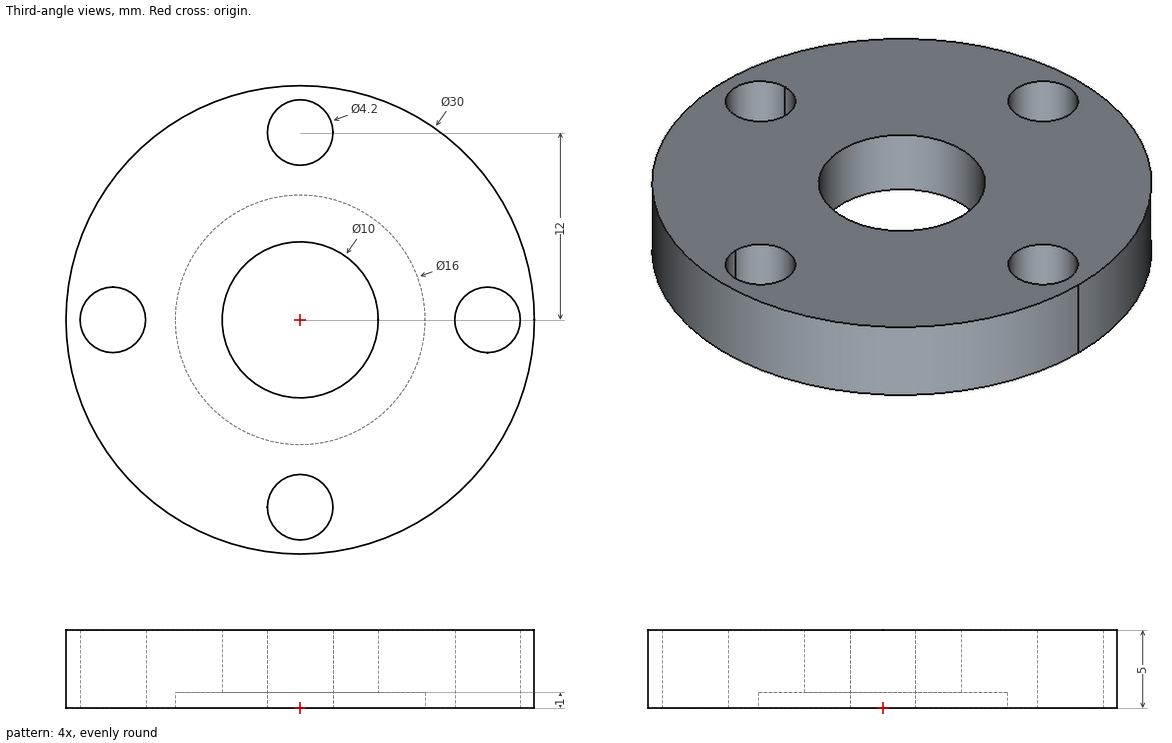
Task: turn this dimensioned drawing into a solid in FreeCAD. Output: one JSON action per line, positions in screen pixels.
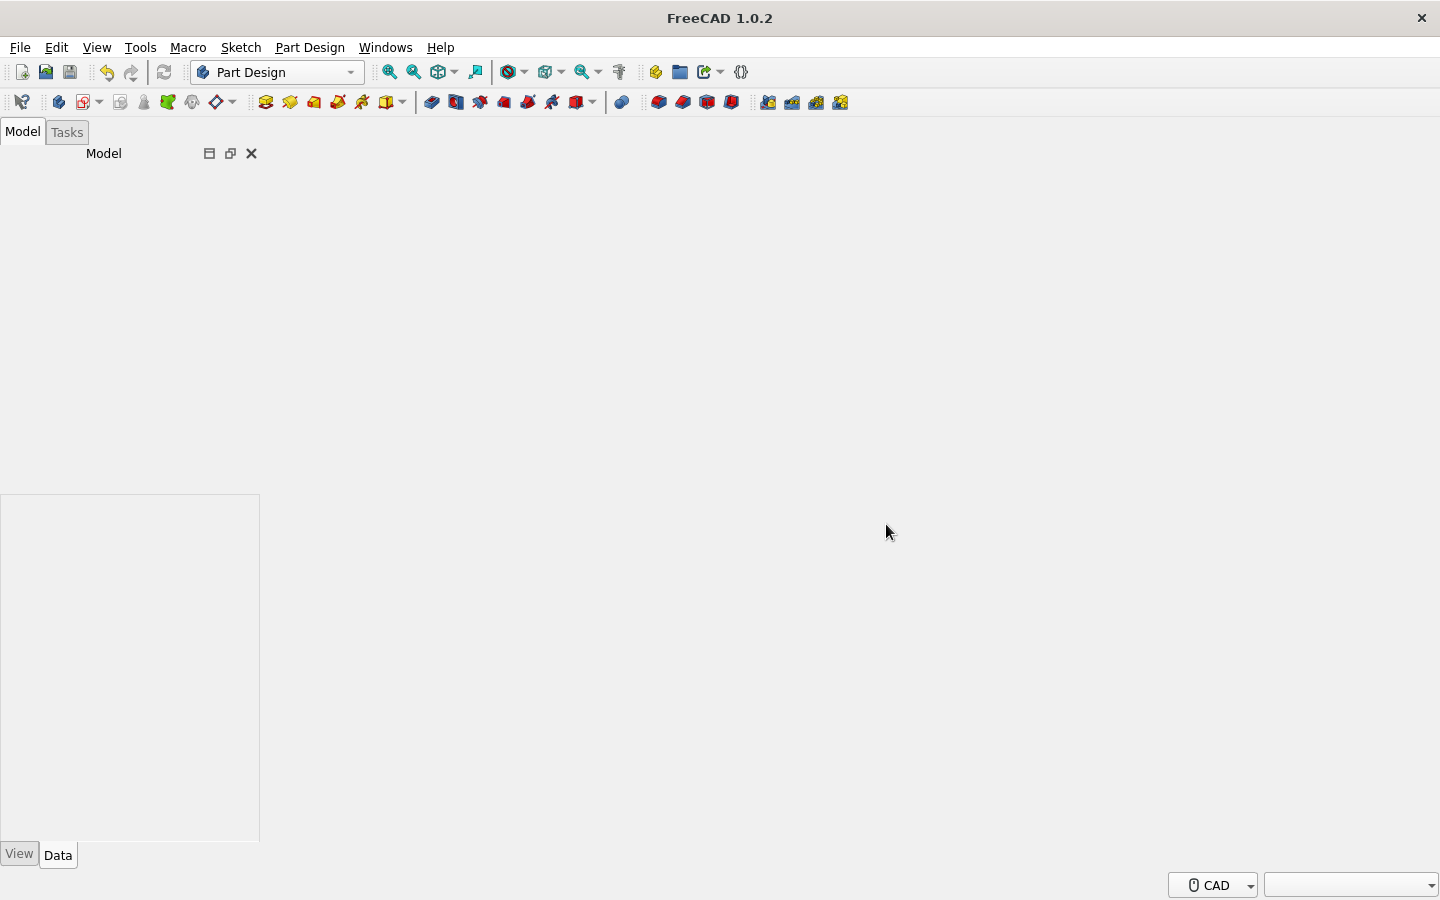
{"action": "left_click", "coordinate": [22, 72]}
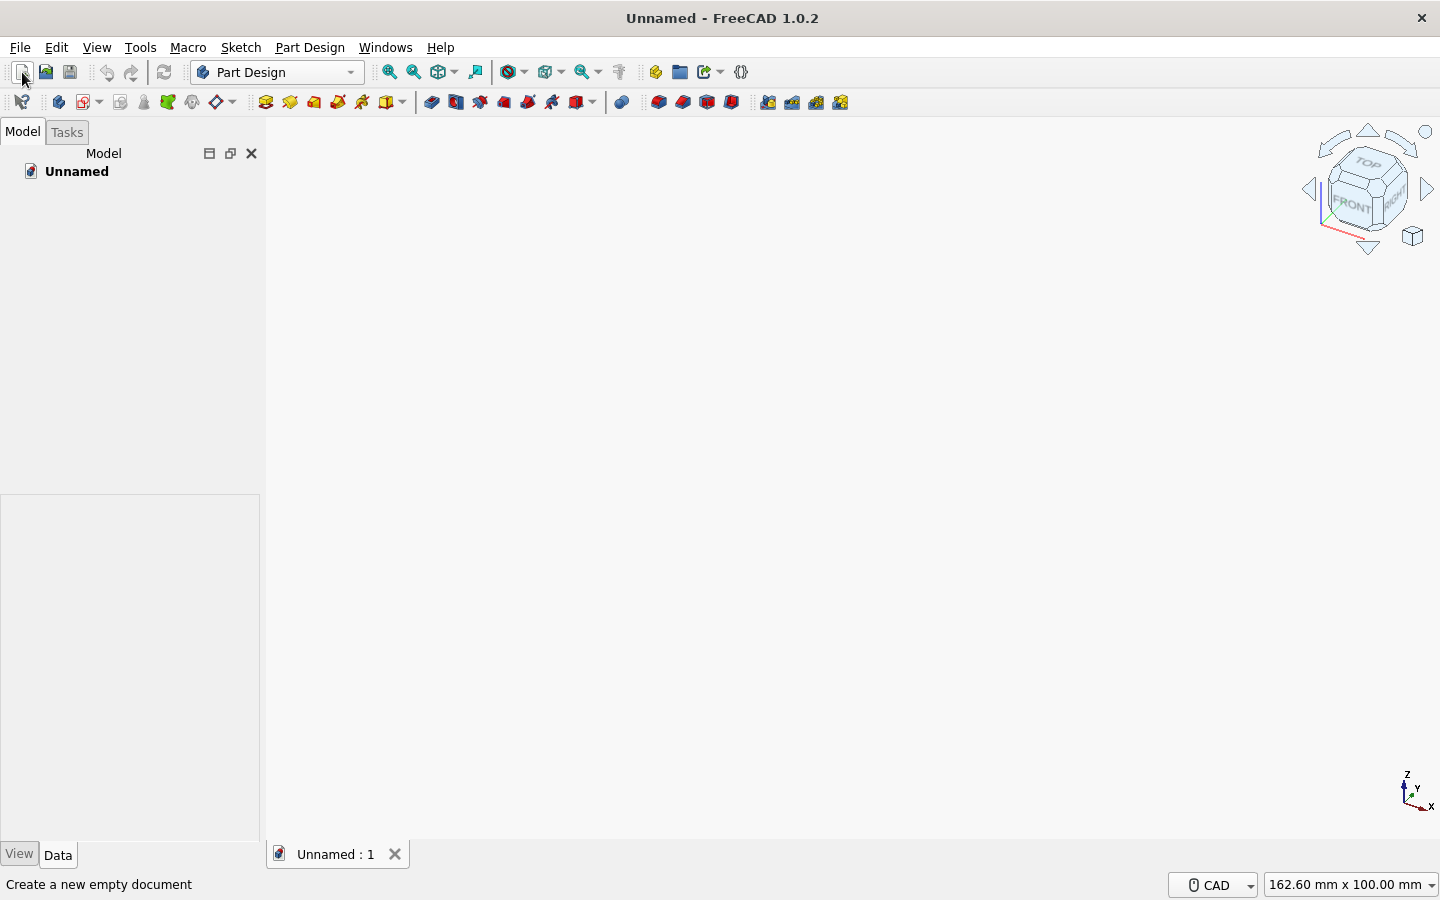
{"action": "left_click", "coordinate": [84, 102]}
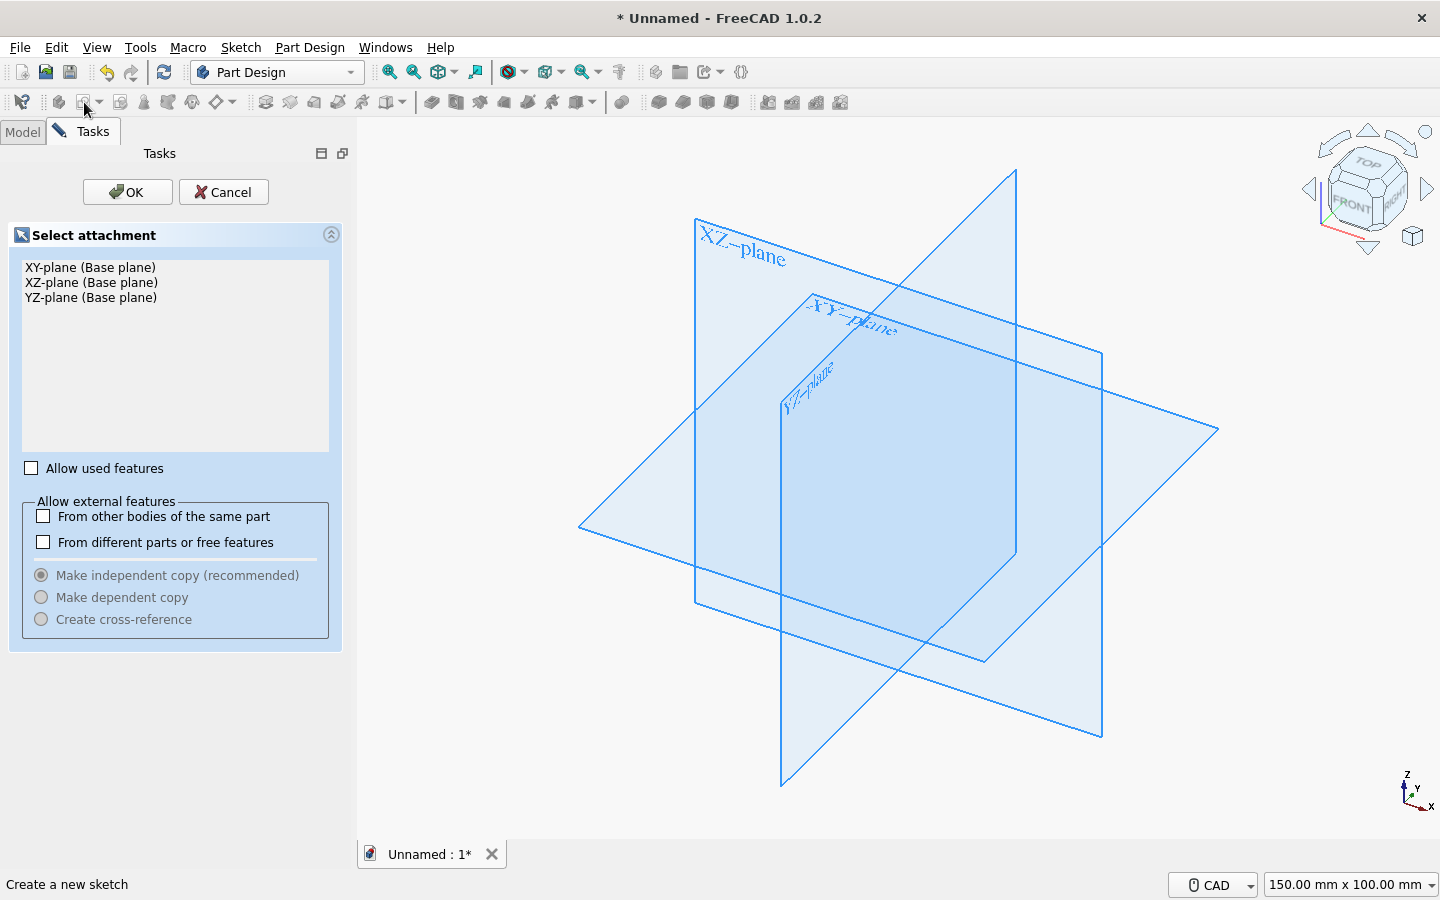
{"action": "left_click", "coordinate": [82, 268]}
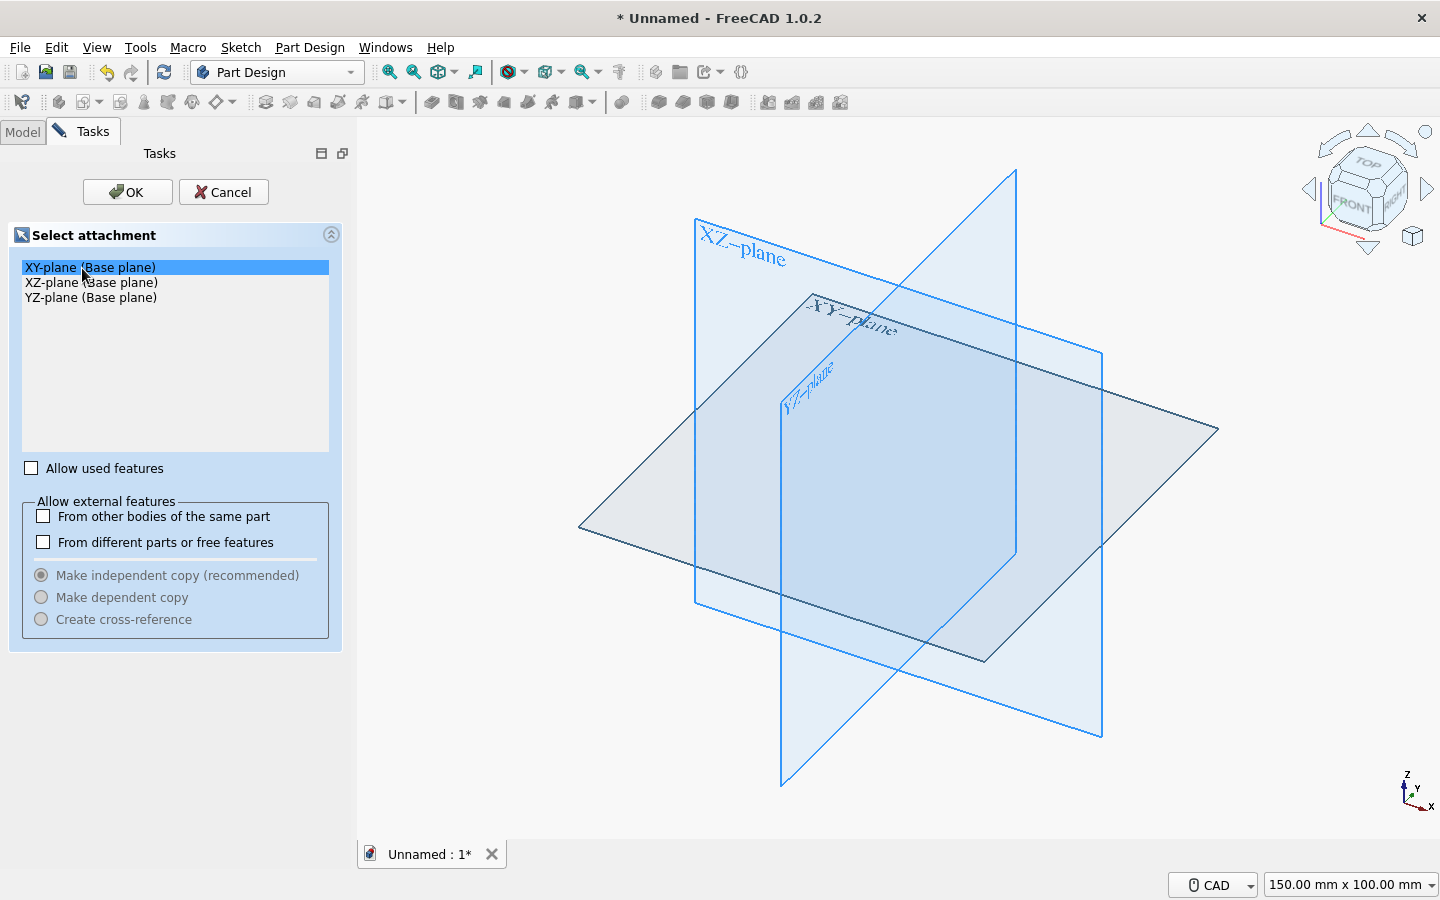
{"action": "left_click", "coordinate": [128, 192]}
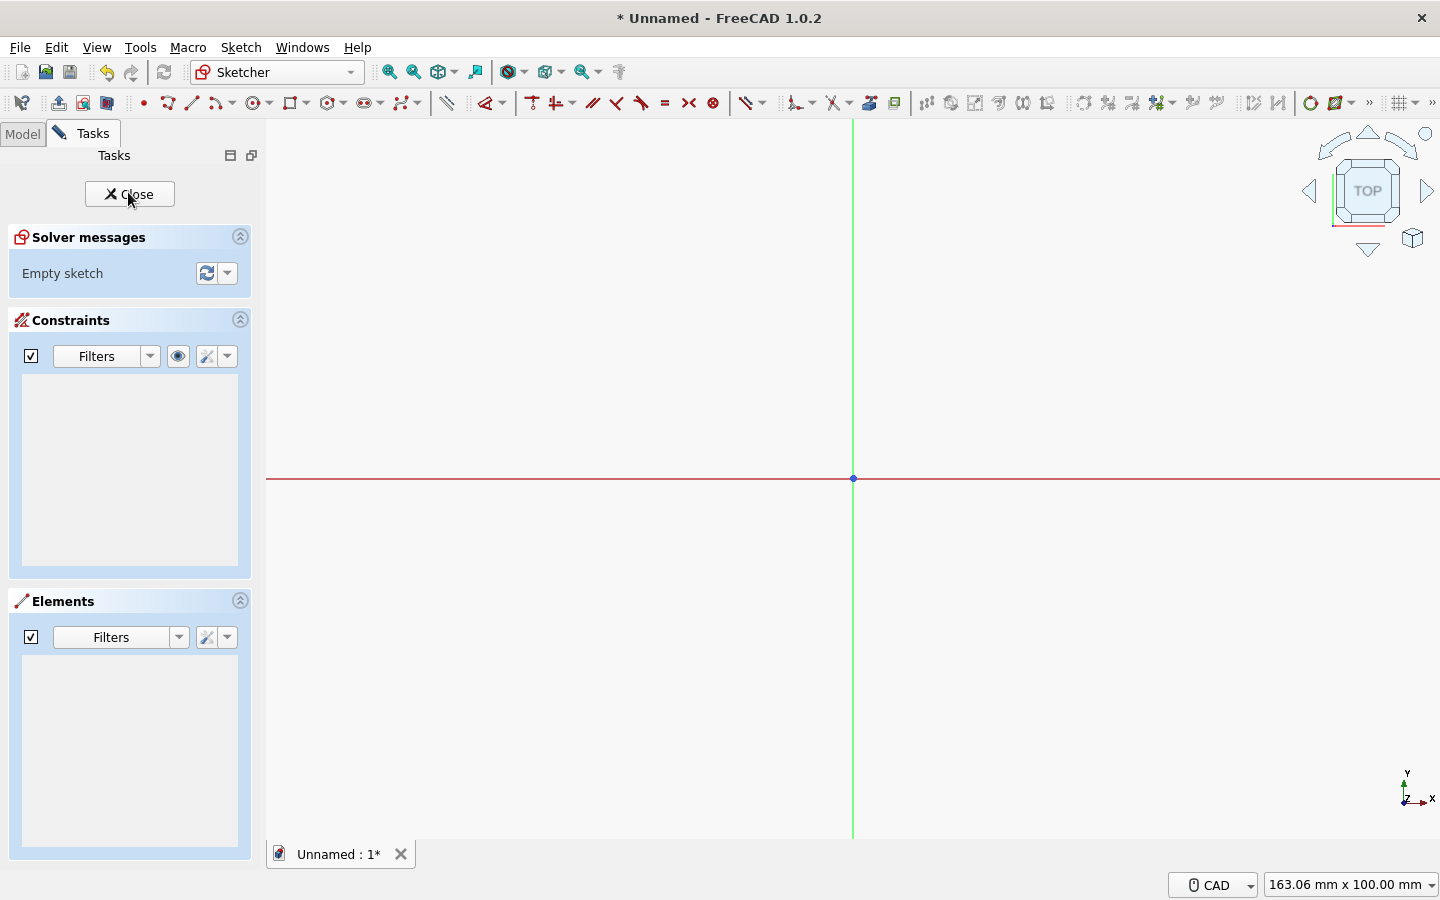
{"action": "scroll", "coordinate": [909, 479], "scroll_direction": "up", "scroll_amount": 4}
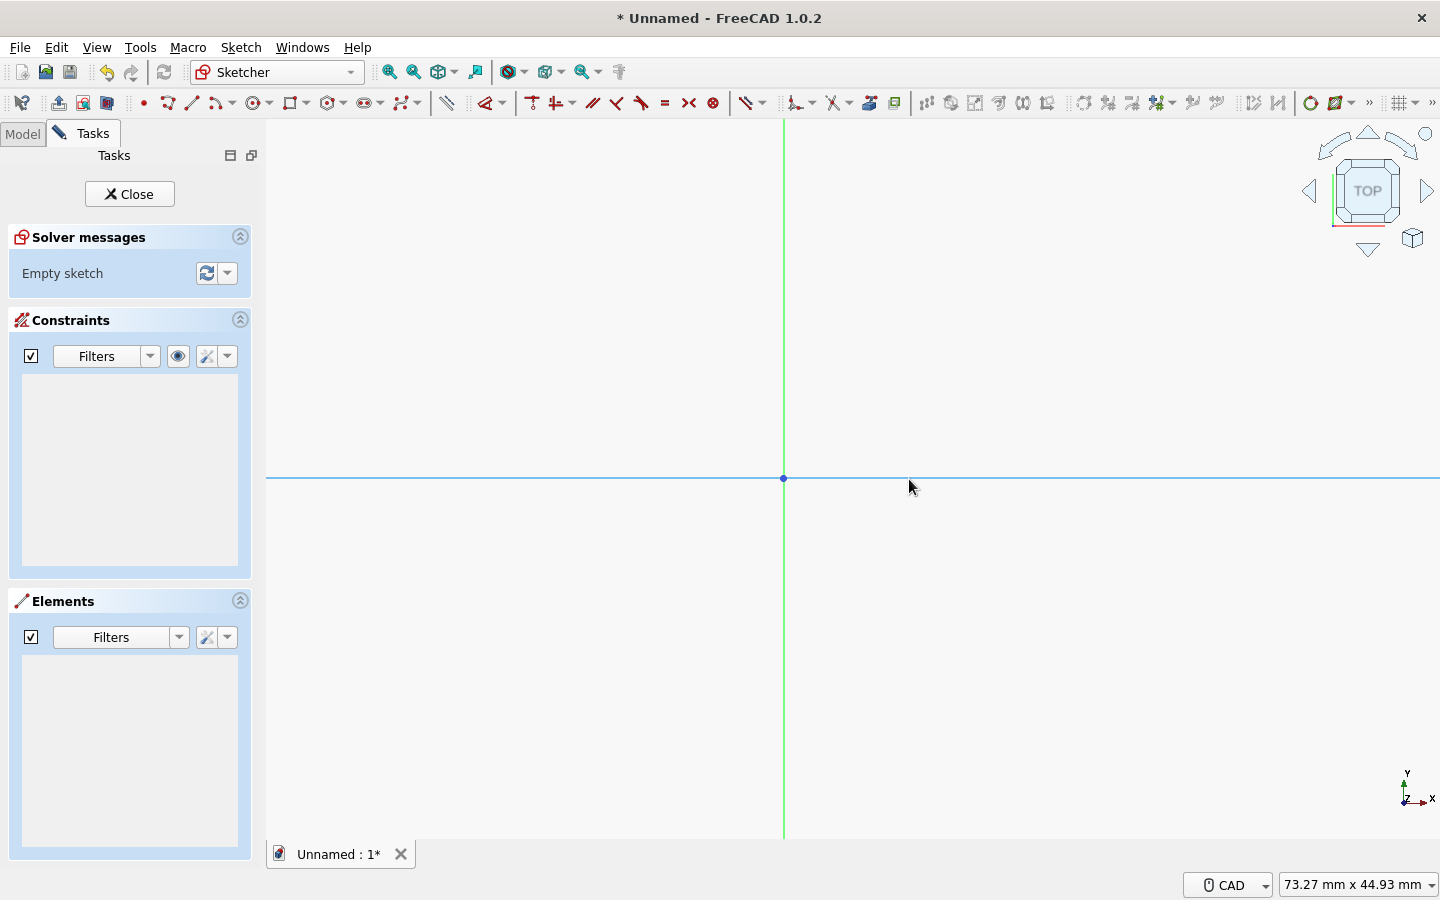
{"action": "left_click", "coordinate": [254, 104]}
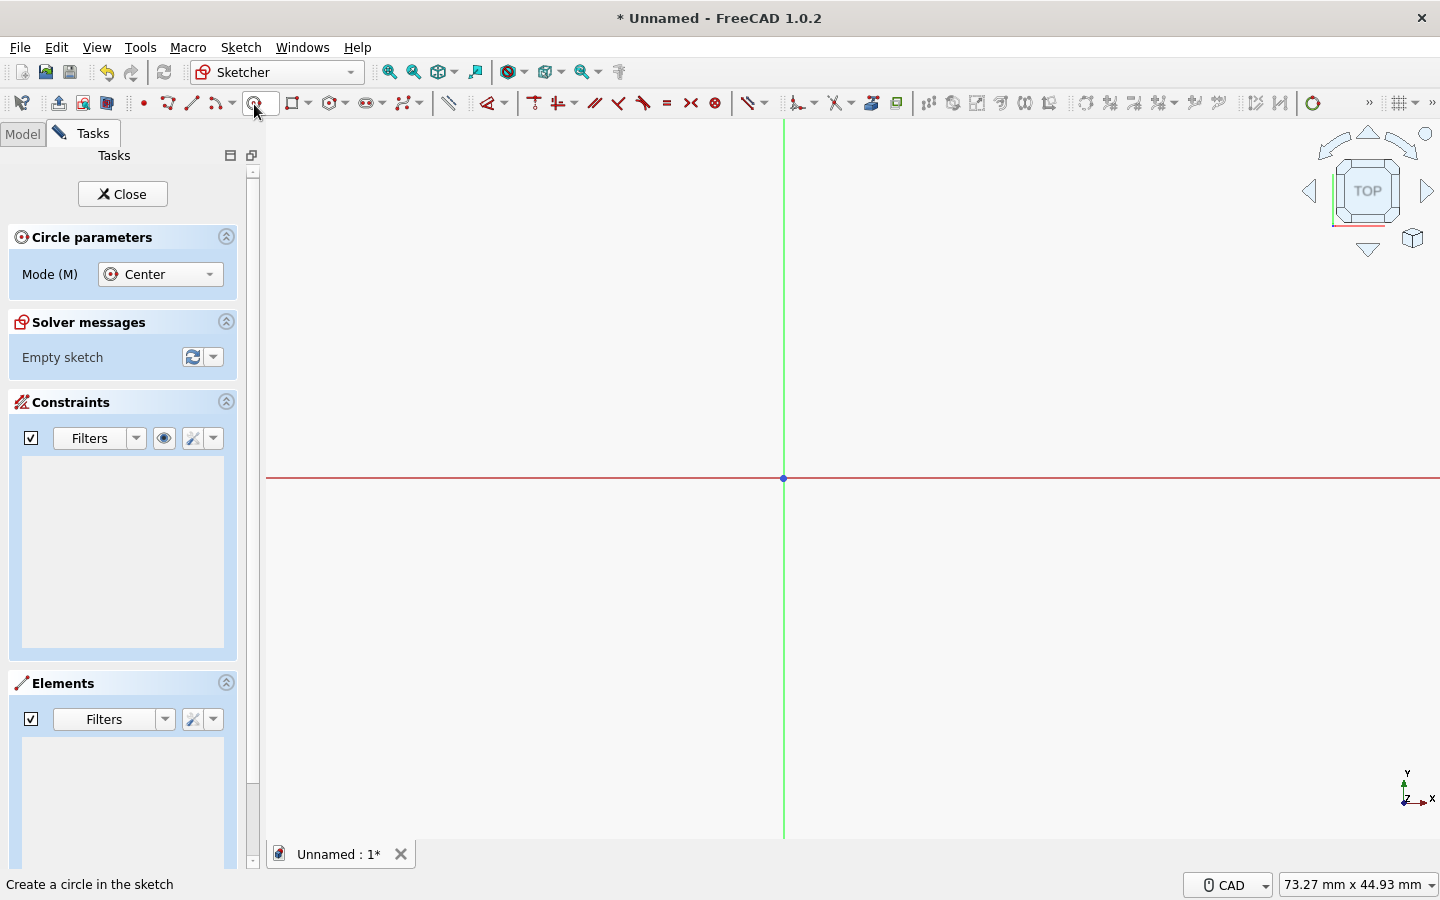
{"action": "left_click", "coordinate": [784, 478]}
{"action": "mouse_move", "coordinate": [954, 308]}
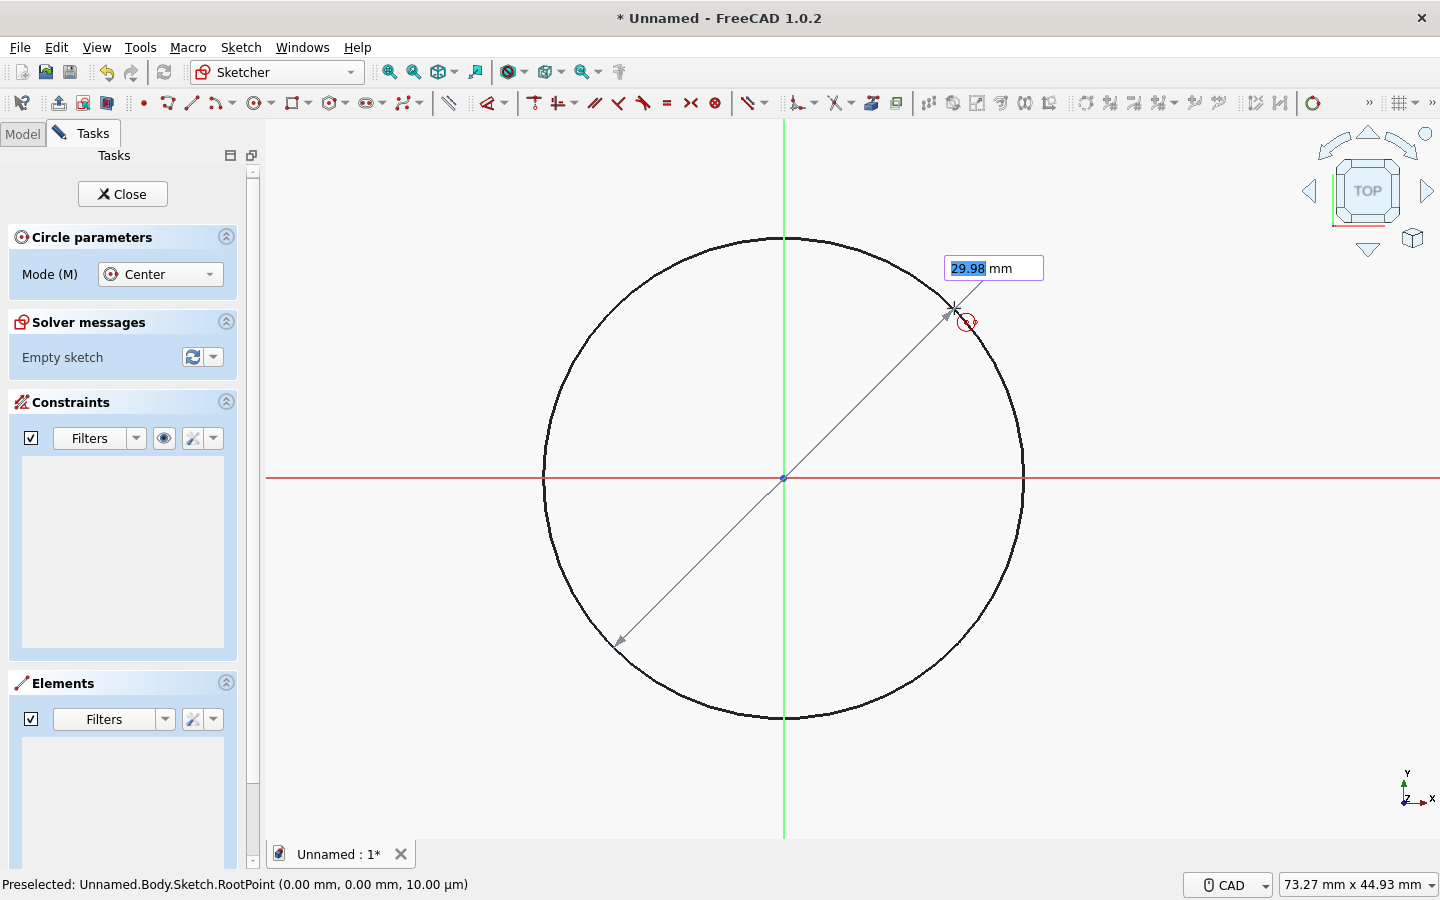
{"action": "type", "text": "30"}
{"action": "key", "text": "Return"}
{"action": "key", "text": "Escape"}